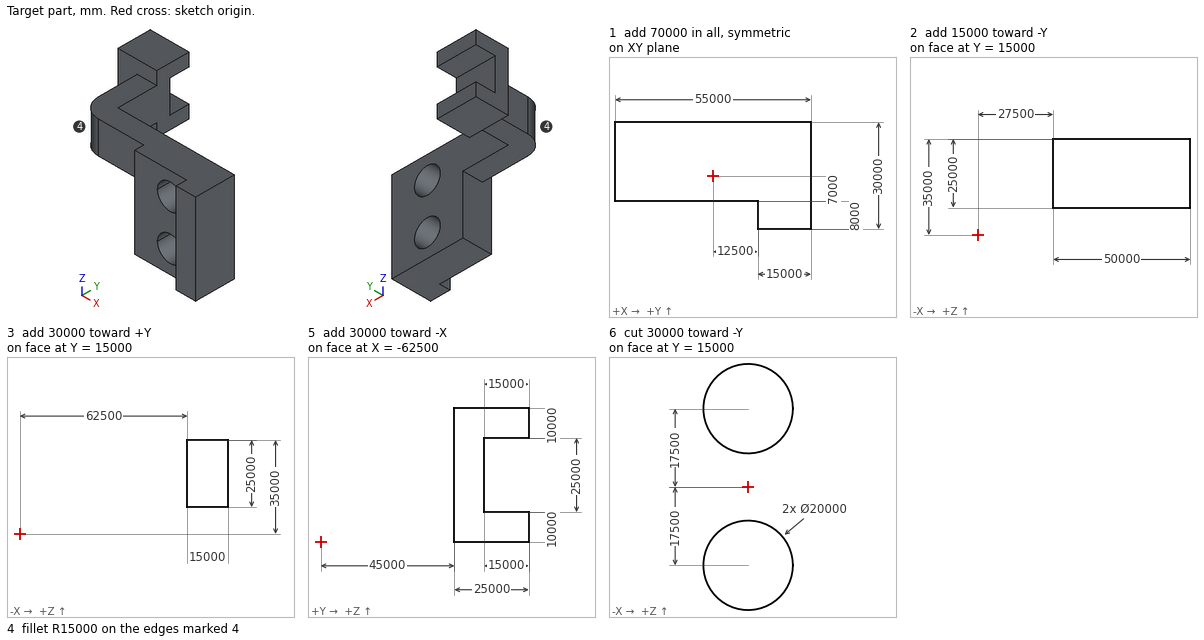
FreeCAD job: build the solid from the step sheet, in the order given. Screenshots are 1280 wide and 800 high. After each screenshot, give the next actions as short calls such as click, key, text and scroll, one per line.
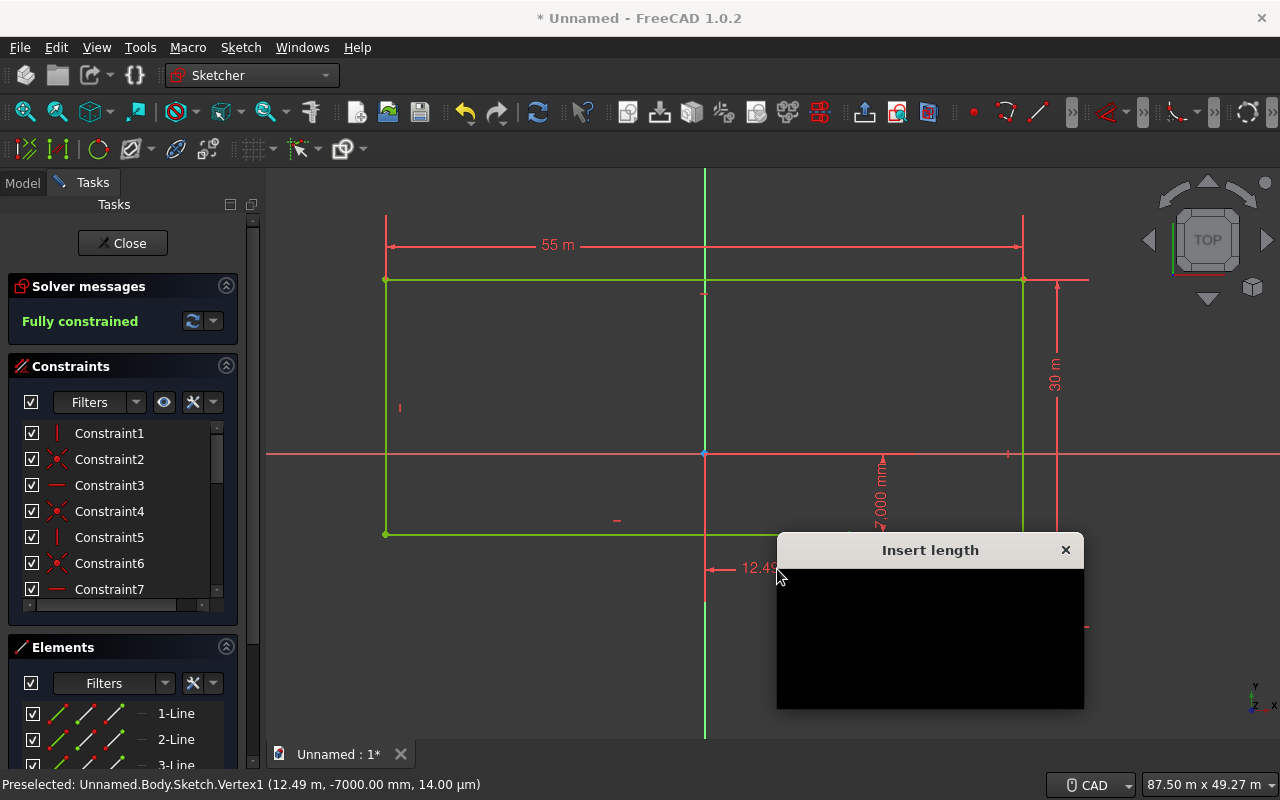
key(ctrl+a)
text(12500 mm)
key(Return)
key(Escape)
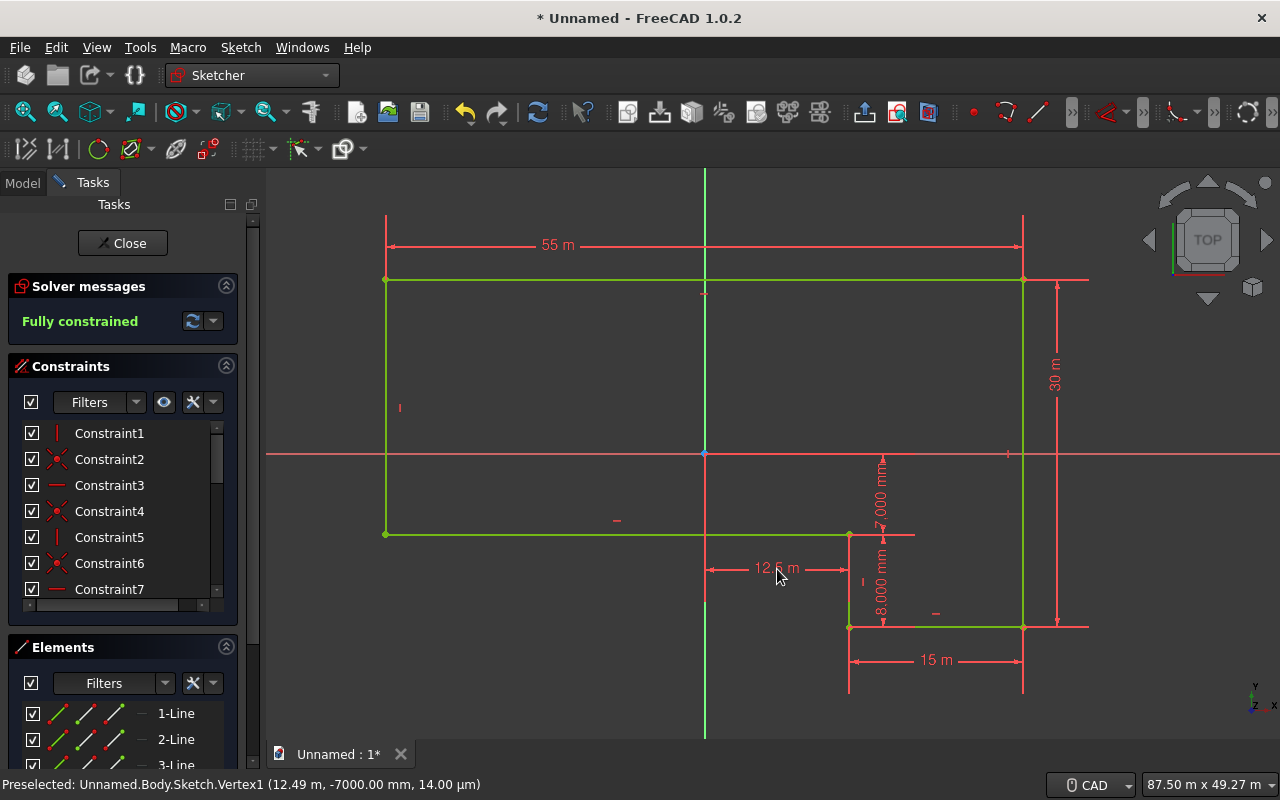
click(123, 243)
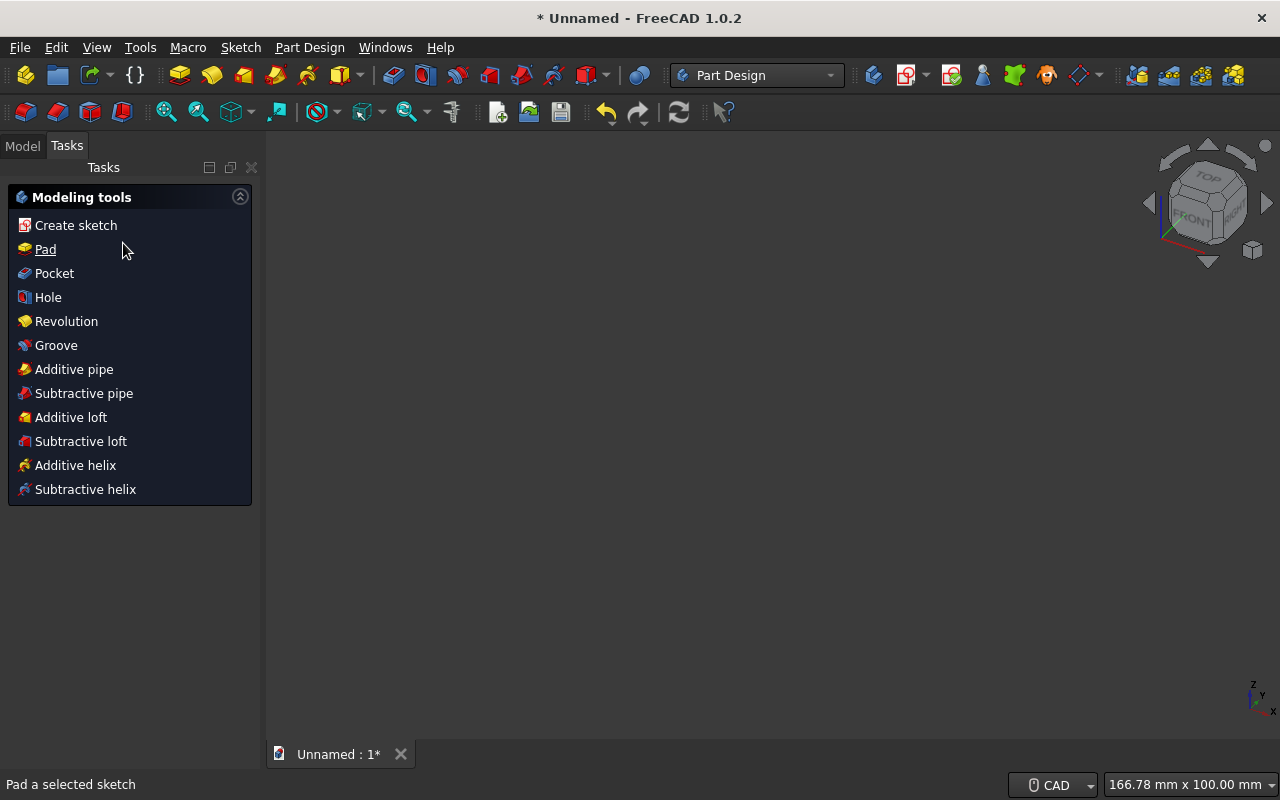
click(180, 76)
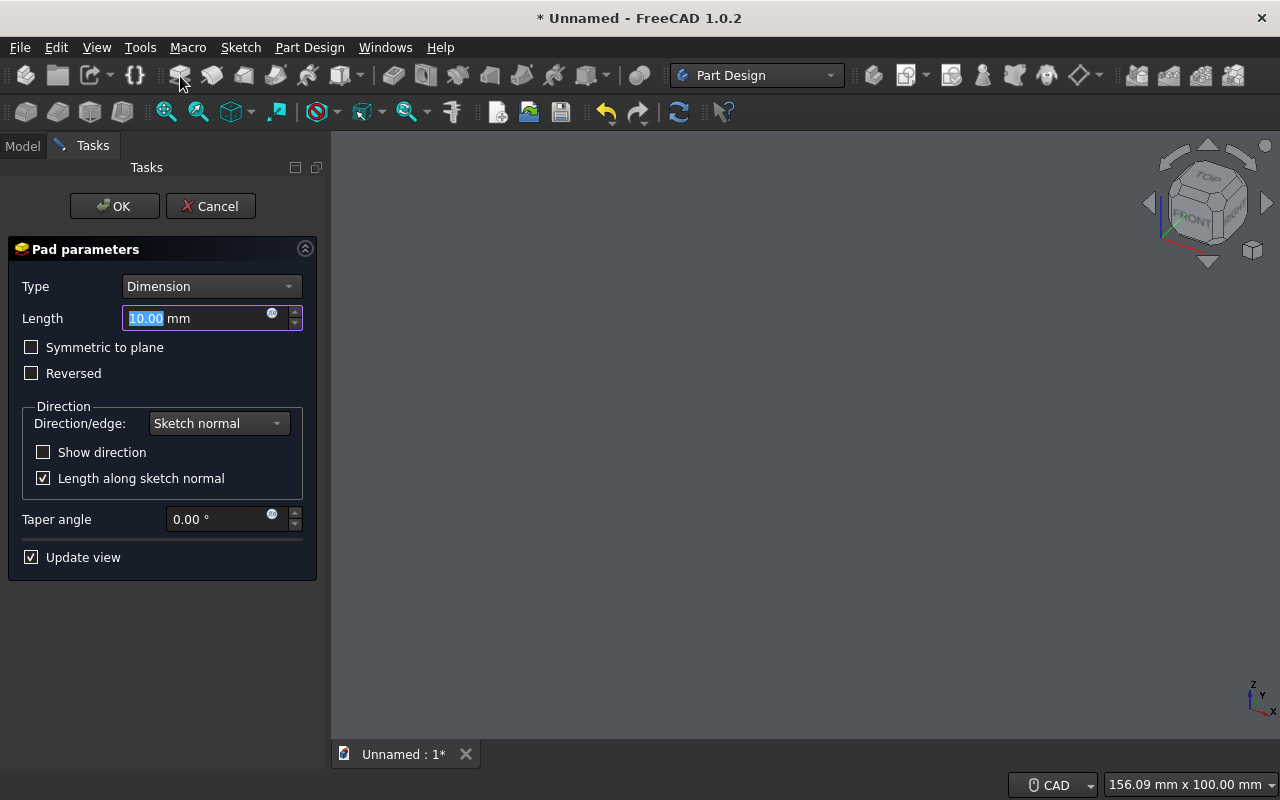
text(70000)
key(Tab)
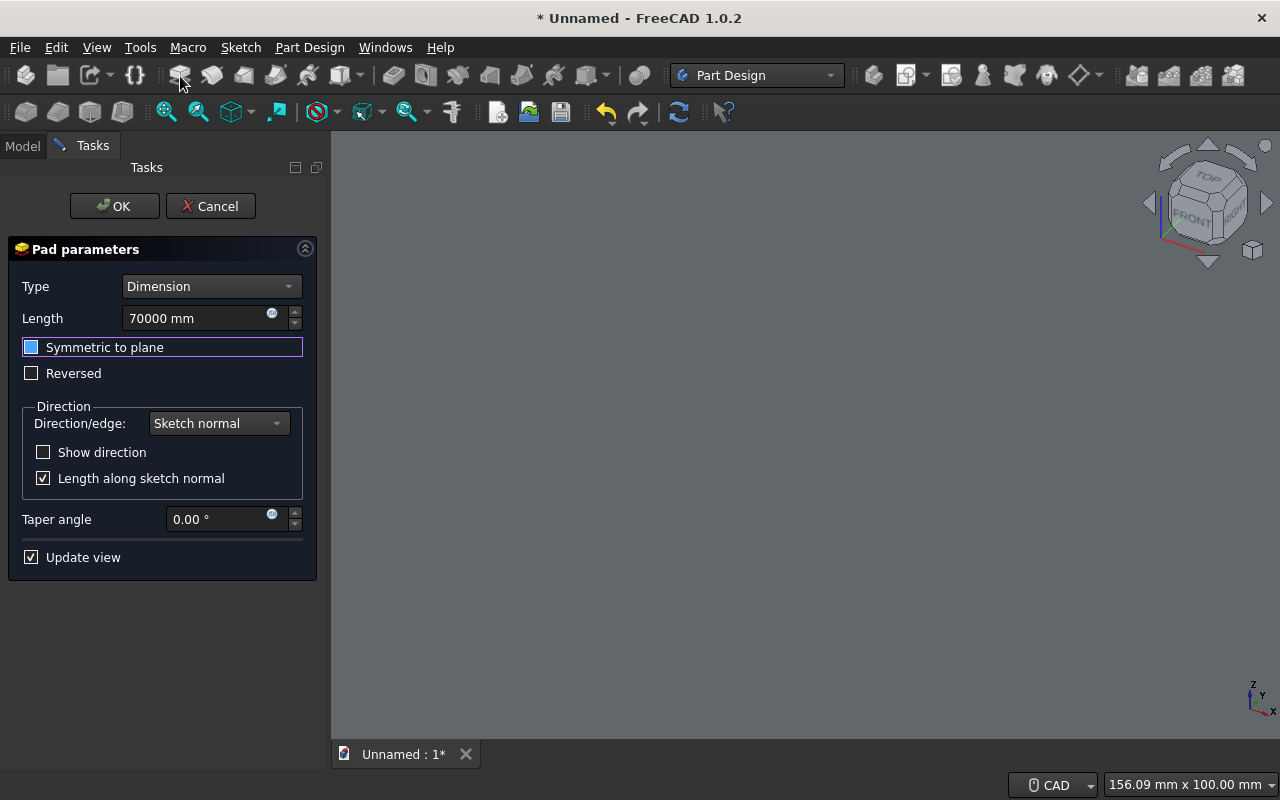
click(30, 347)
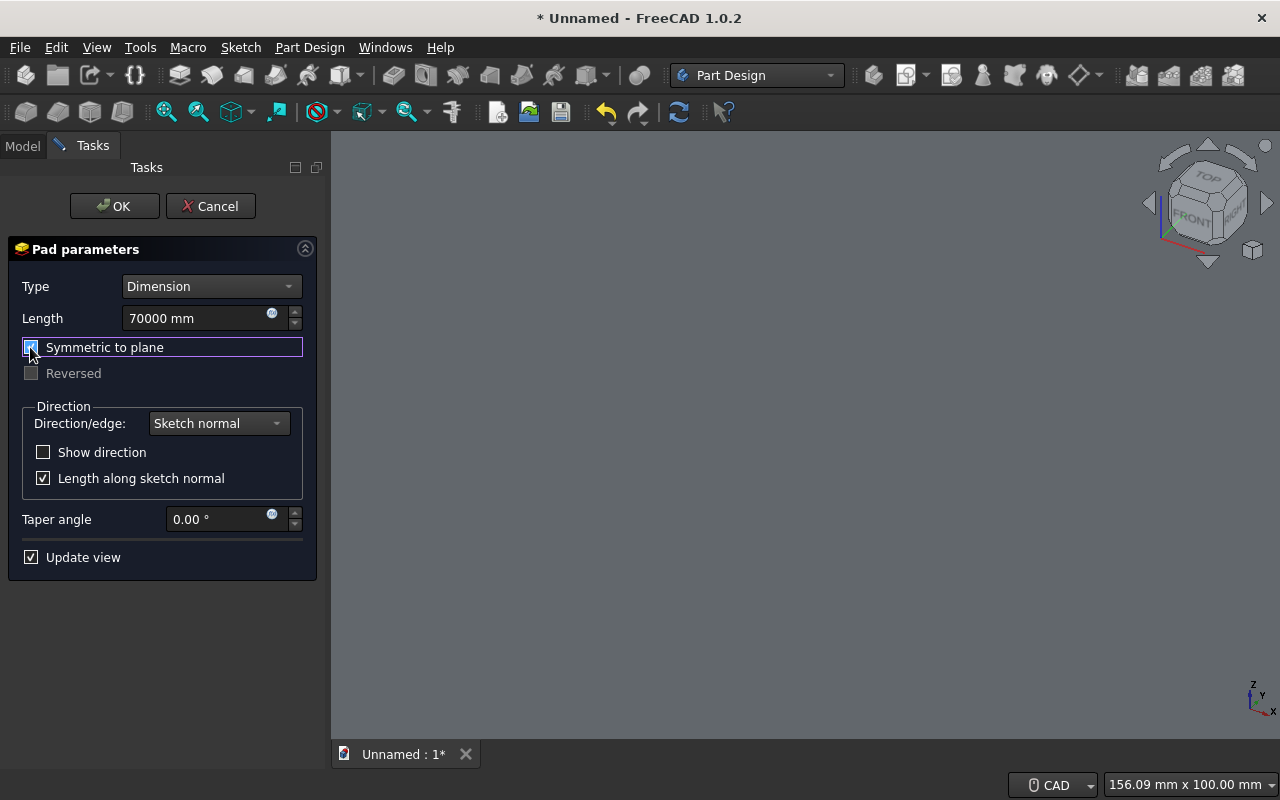
click(115, 206)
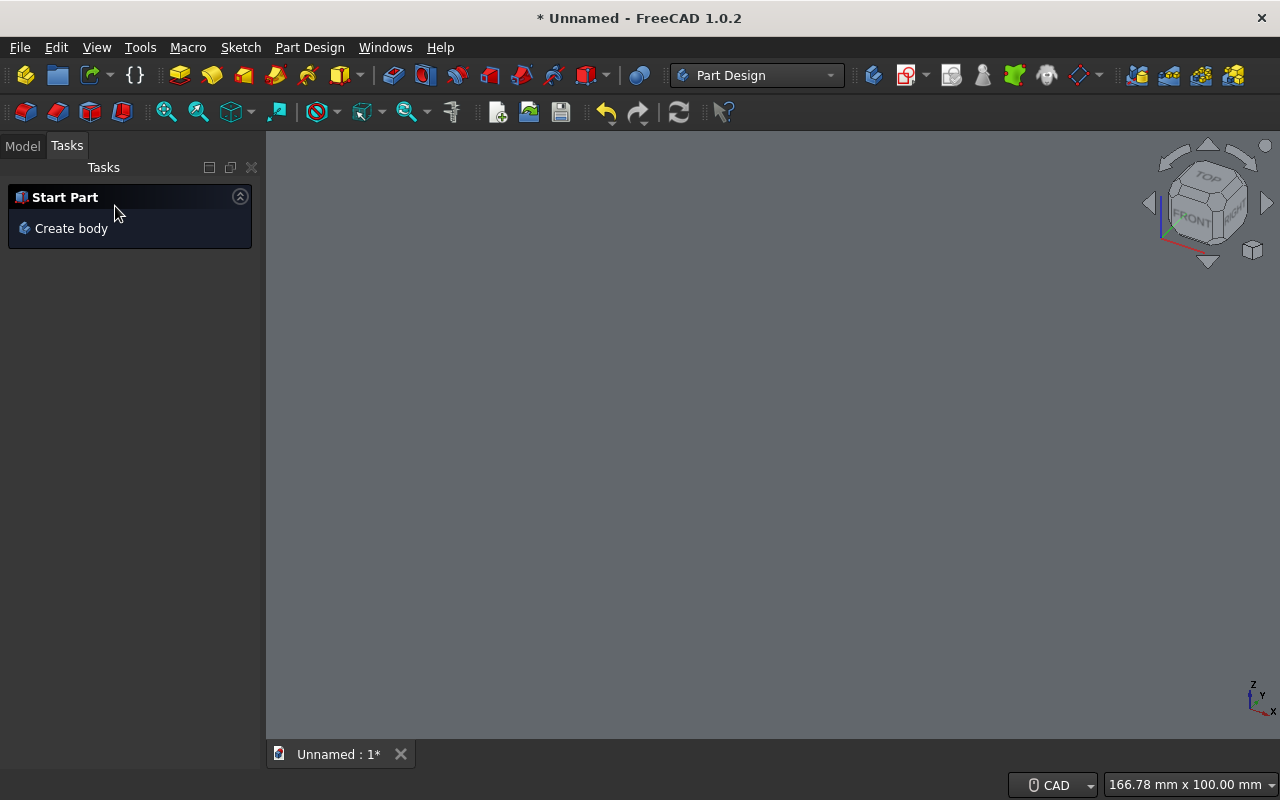
key(v)
key(f)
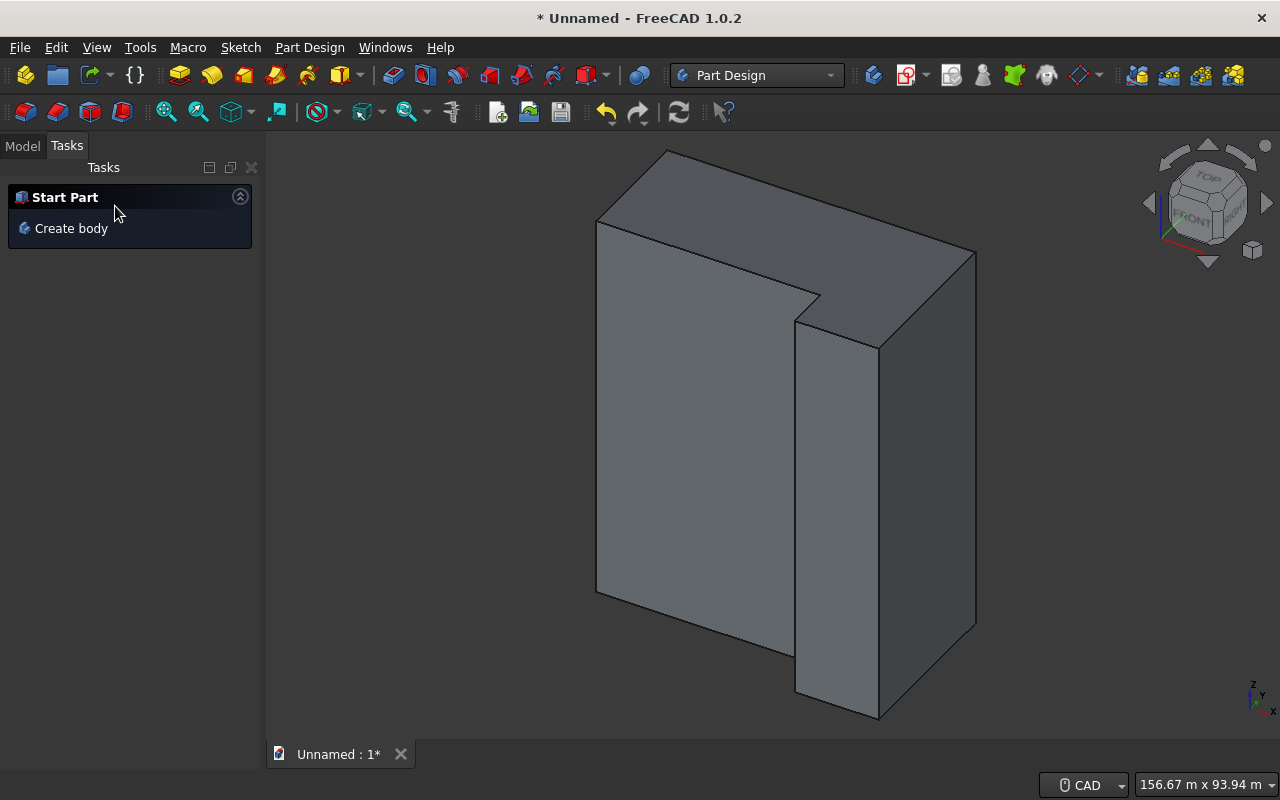
key(4)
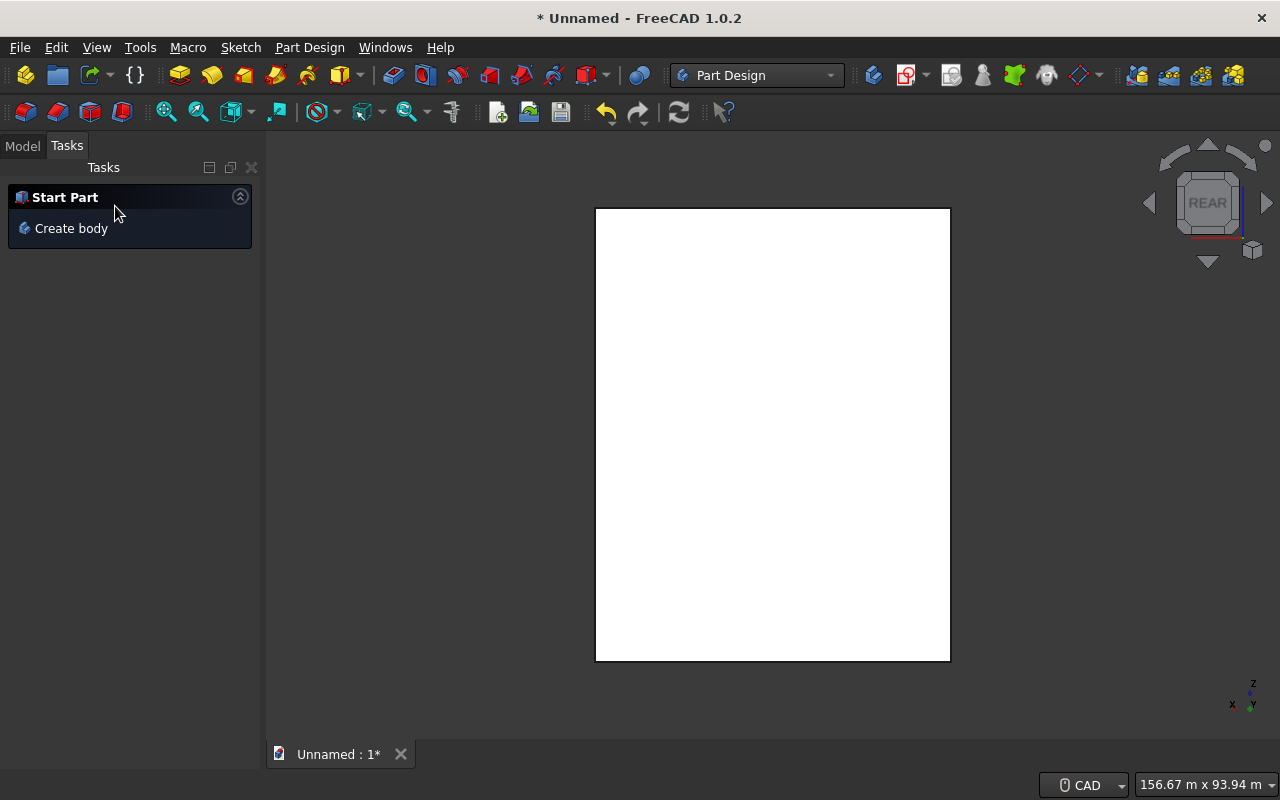
click(773, 434)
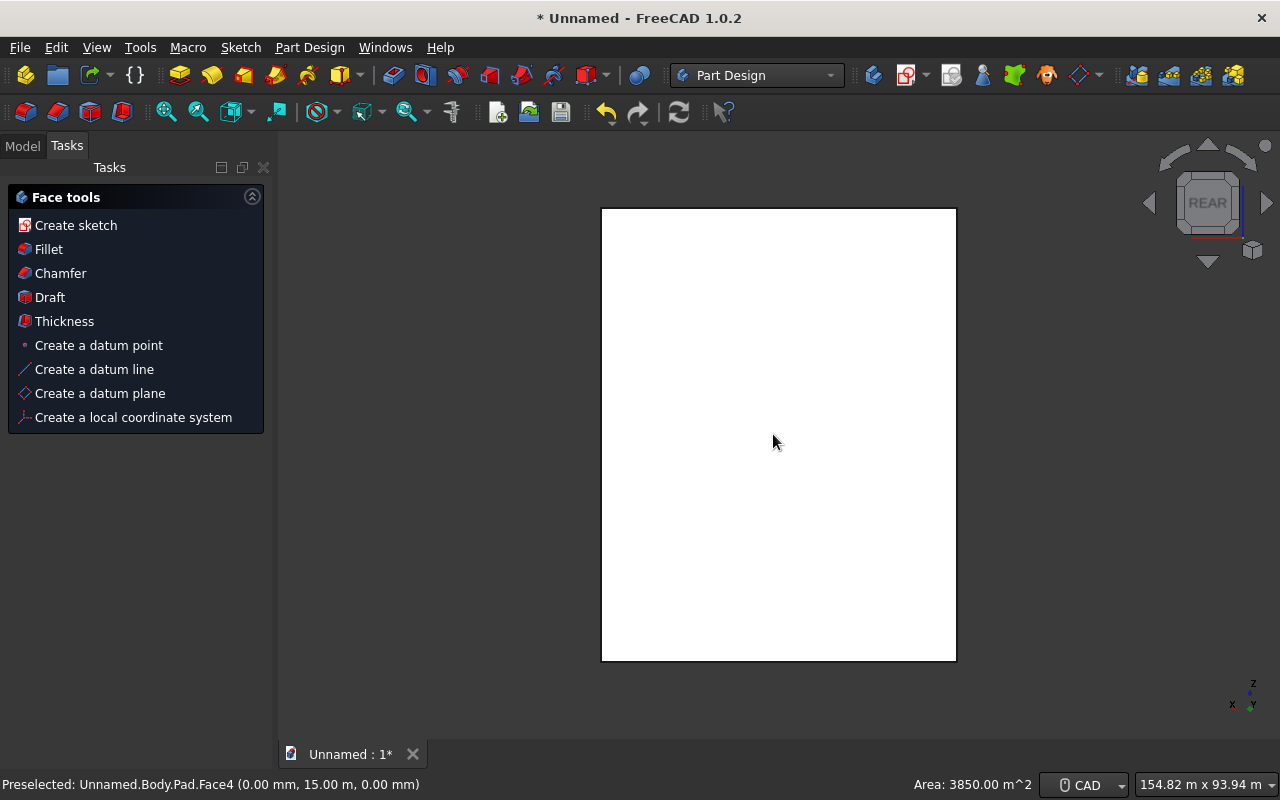
click(906, 76)